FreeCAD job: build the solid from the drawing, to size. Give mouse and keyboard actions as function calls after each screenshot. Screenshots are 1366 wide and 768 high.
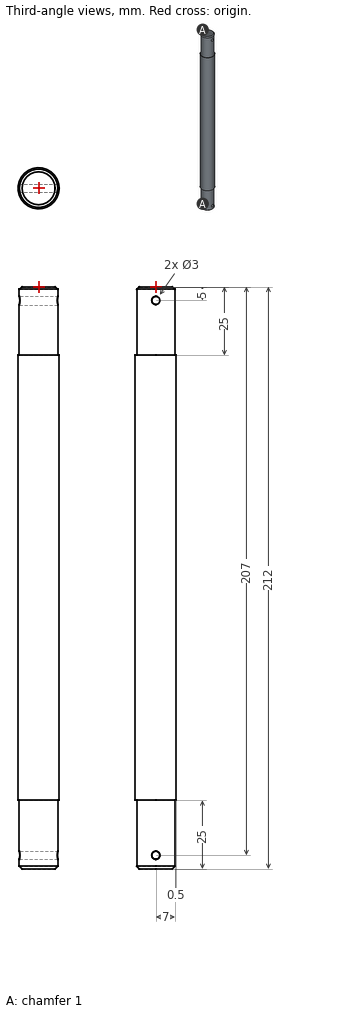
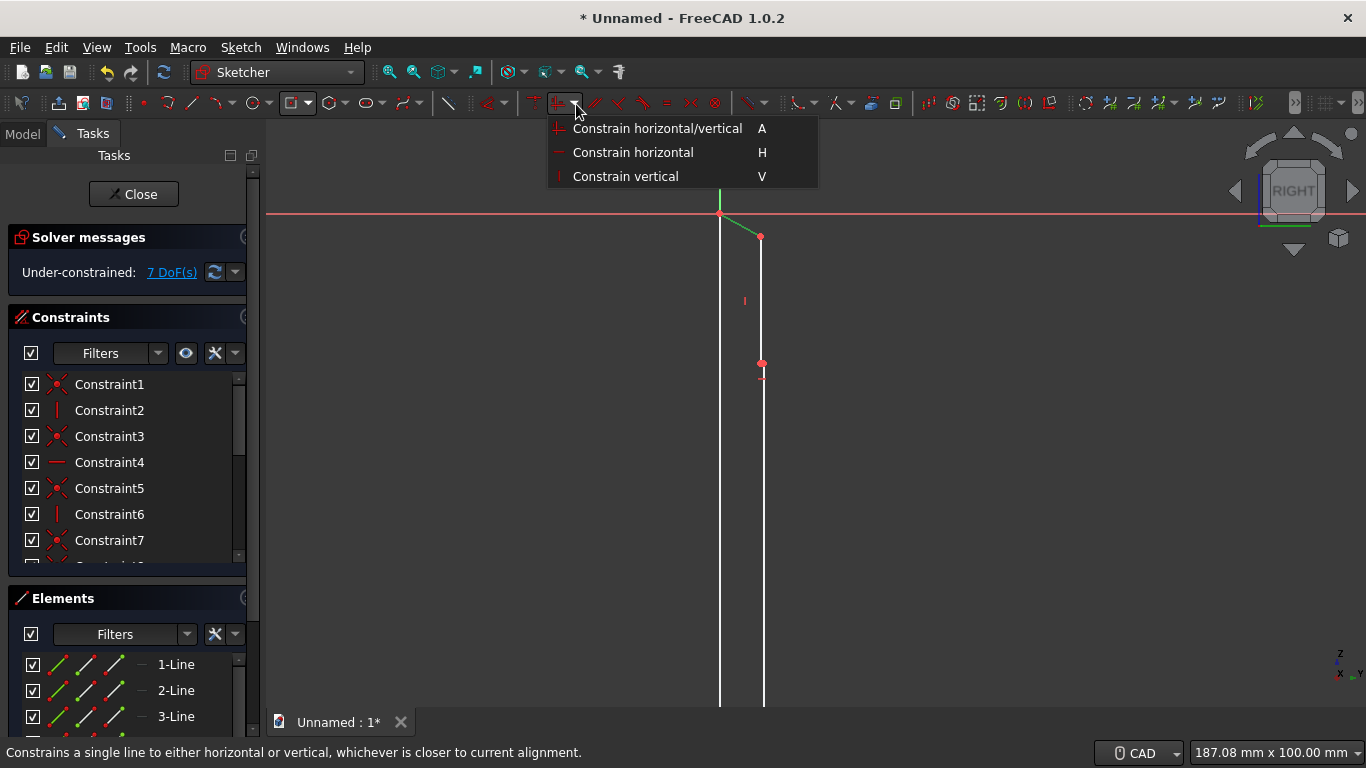
click(683, 152)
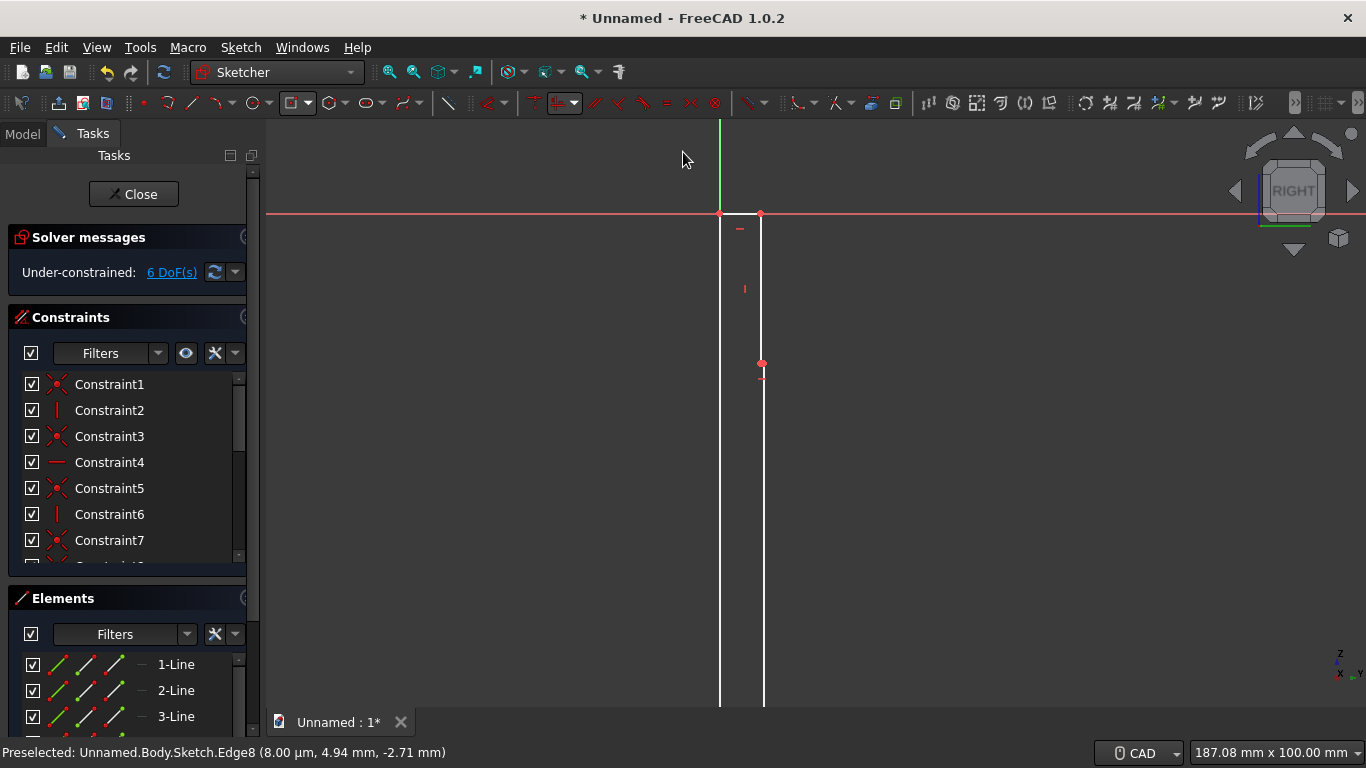
scroll(750, 230, down, 6)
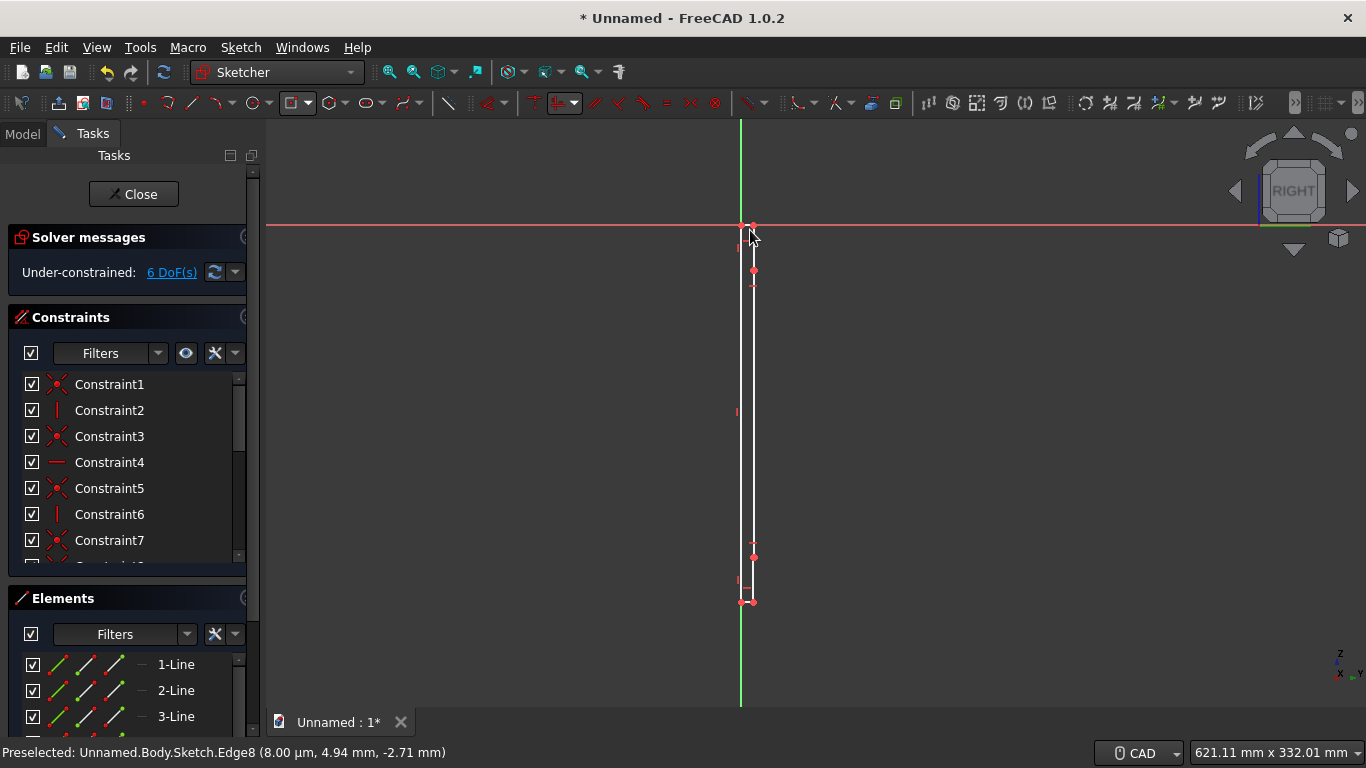
scroll(745, 602, up, 7)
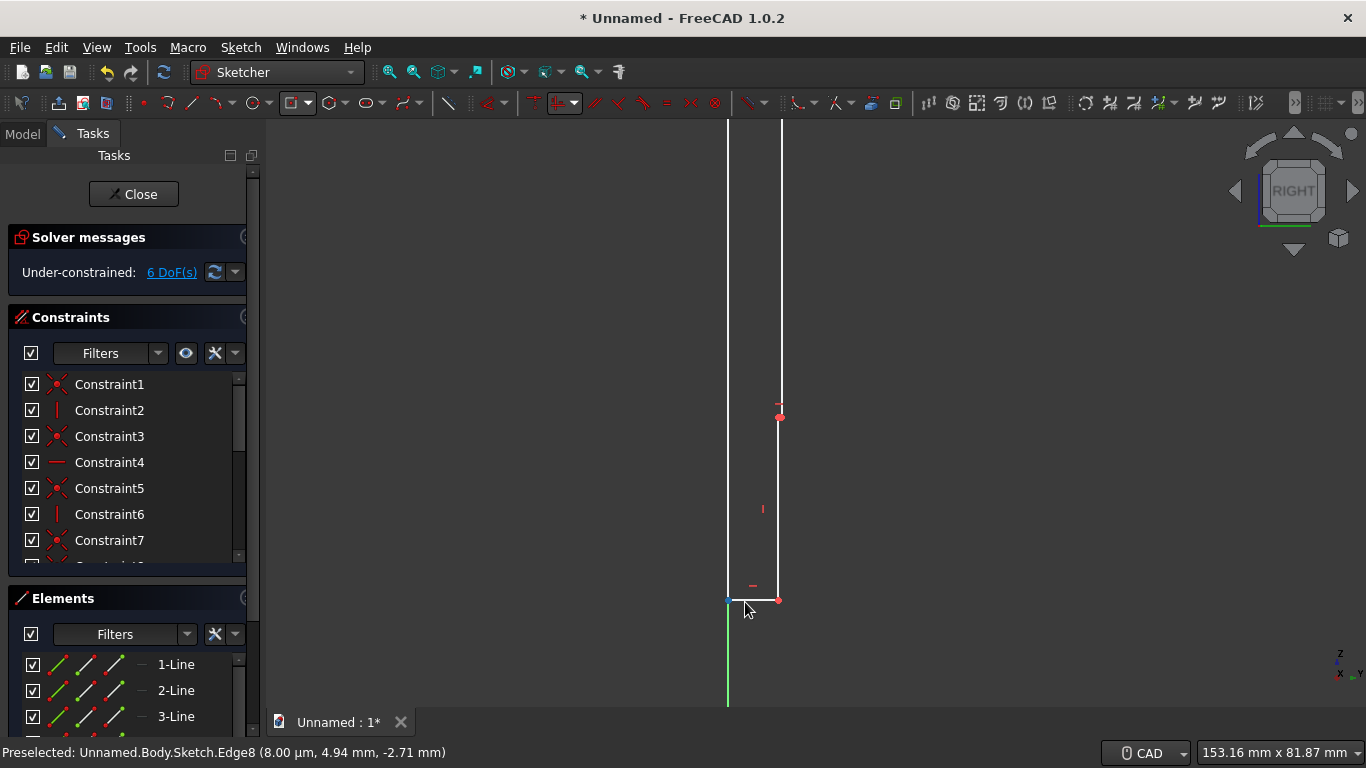
click(743, 600)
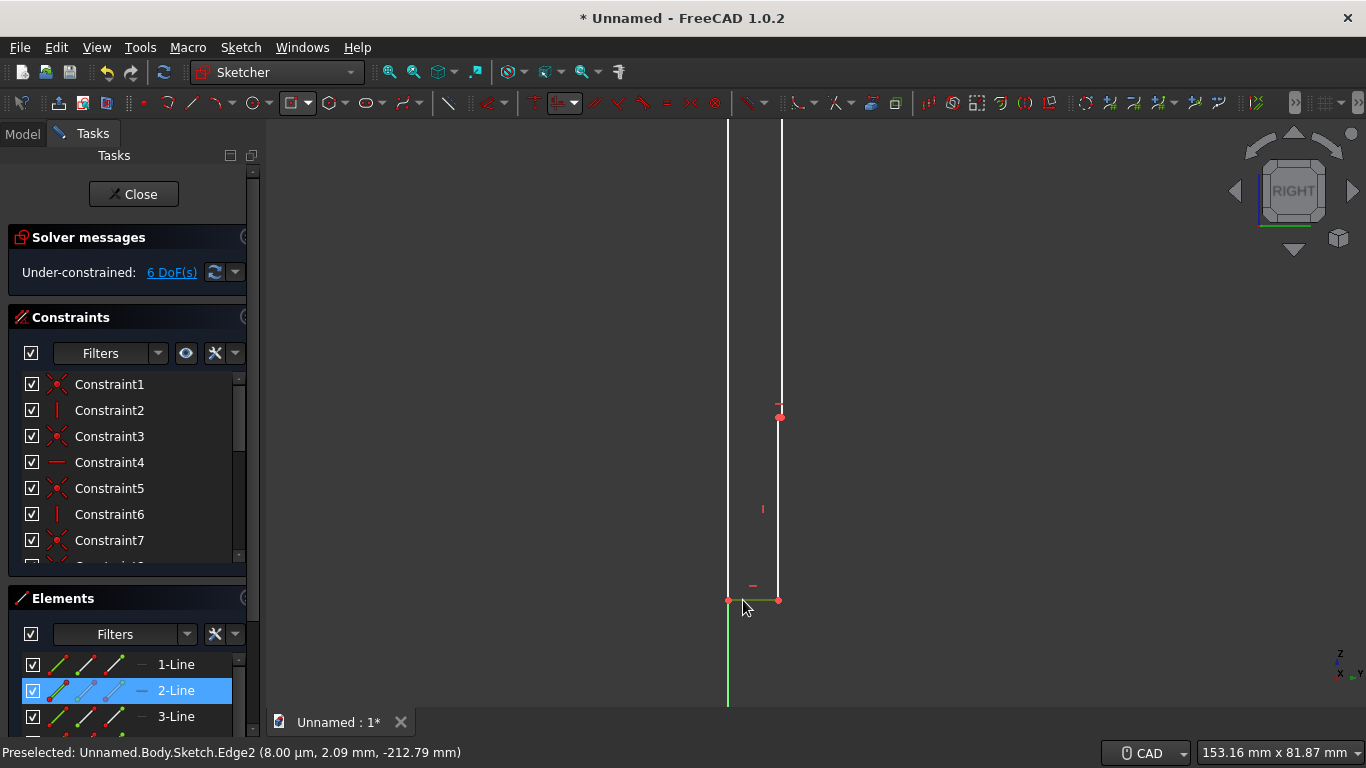
key(l)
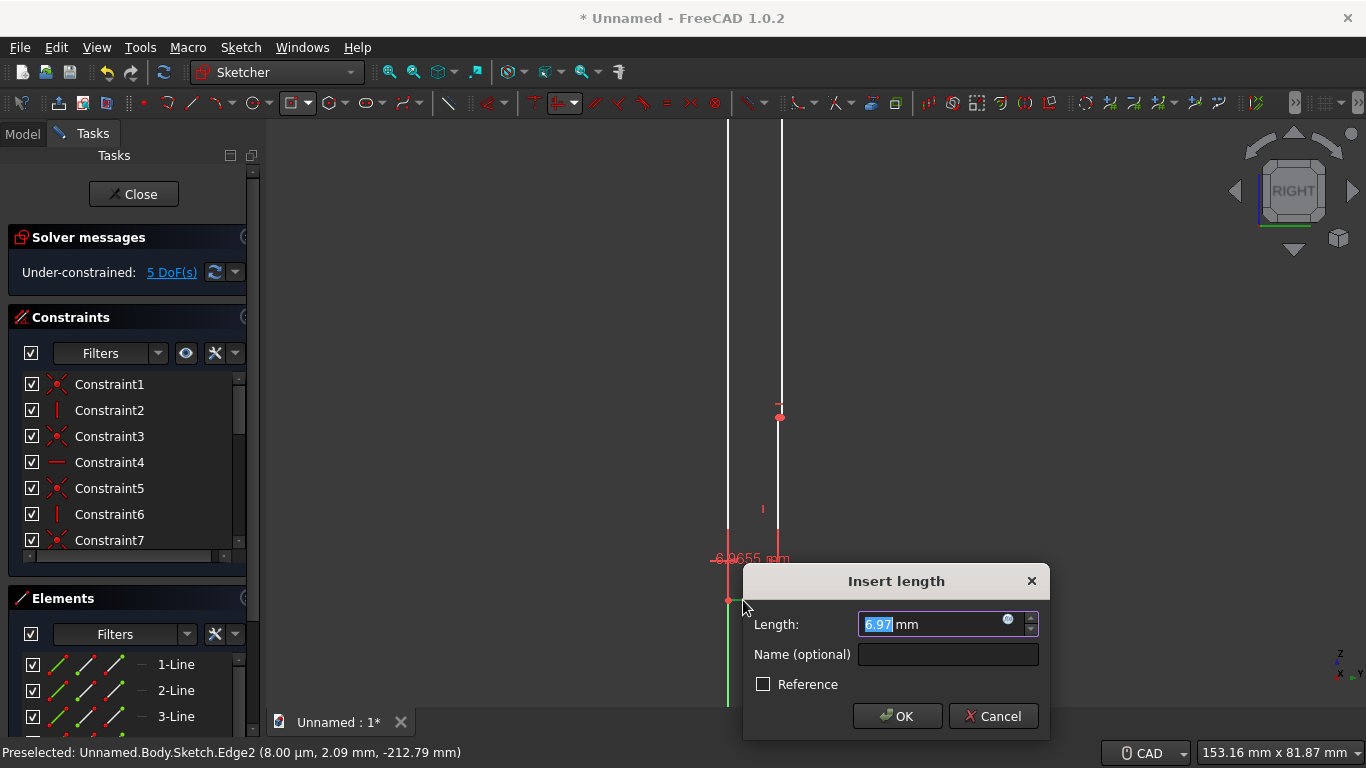
text(7)
key(Return)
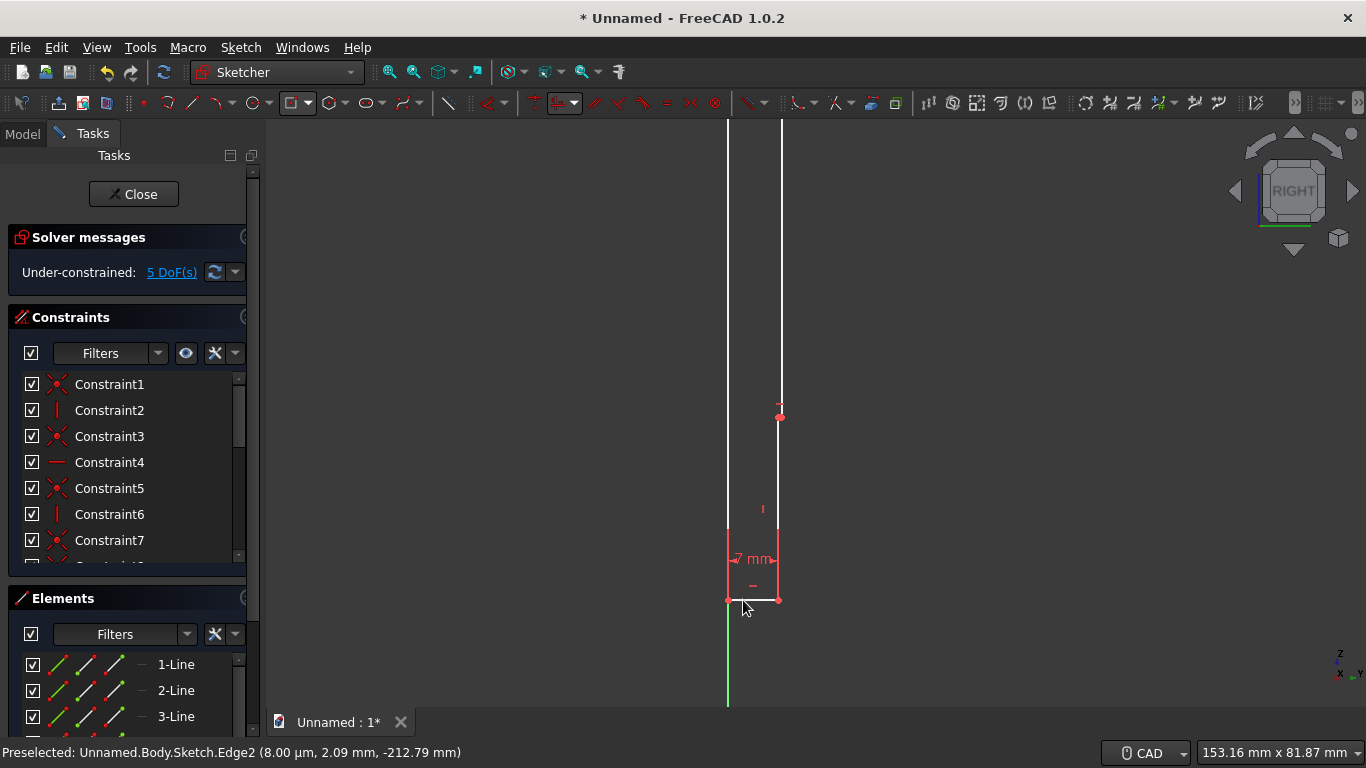
scroll(745, 603, down, 7)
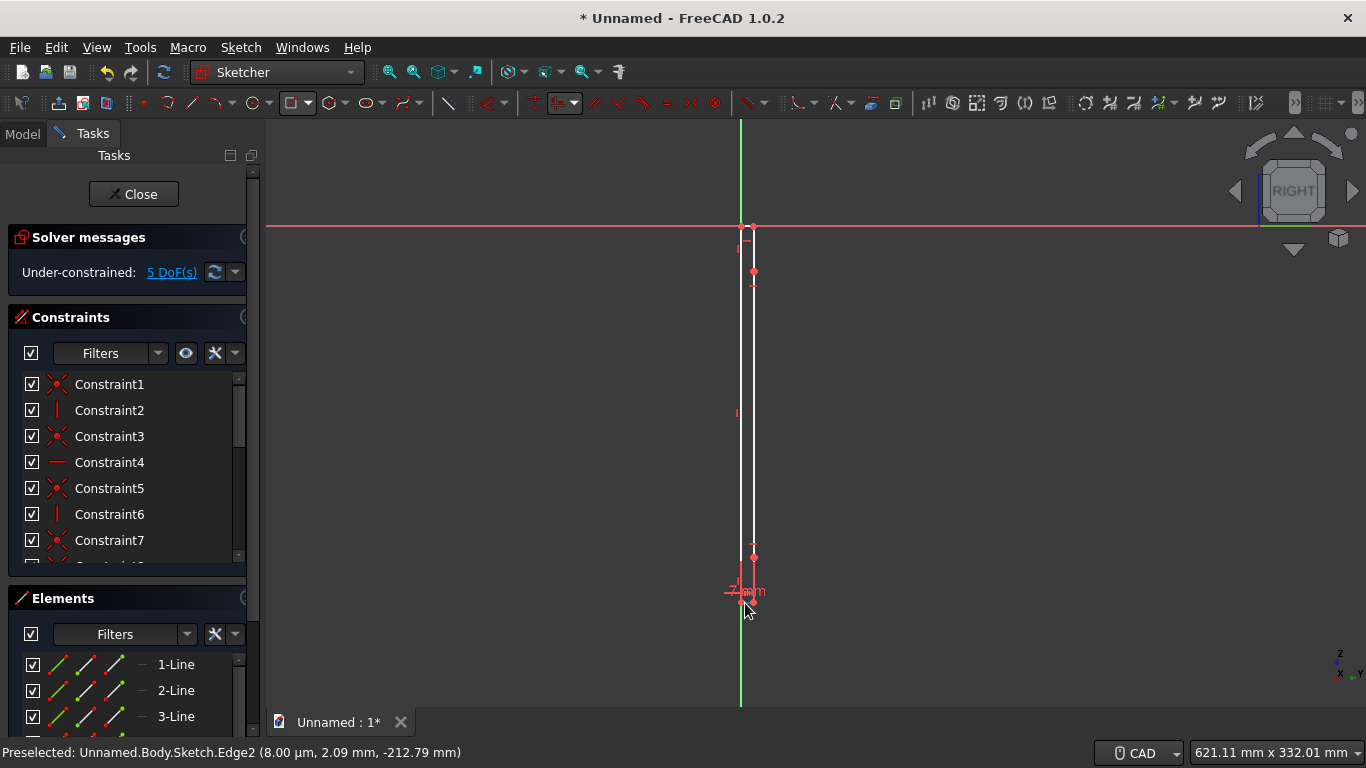
scroll(750, 226, up, 7)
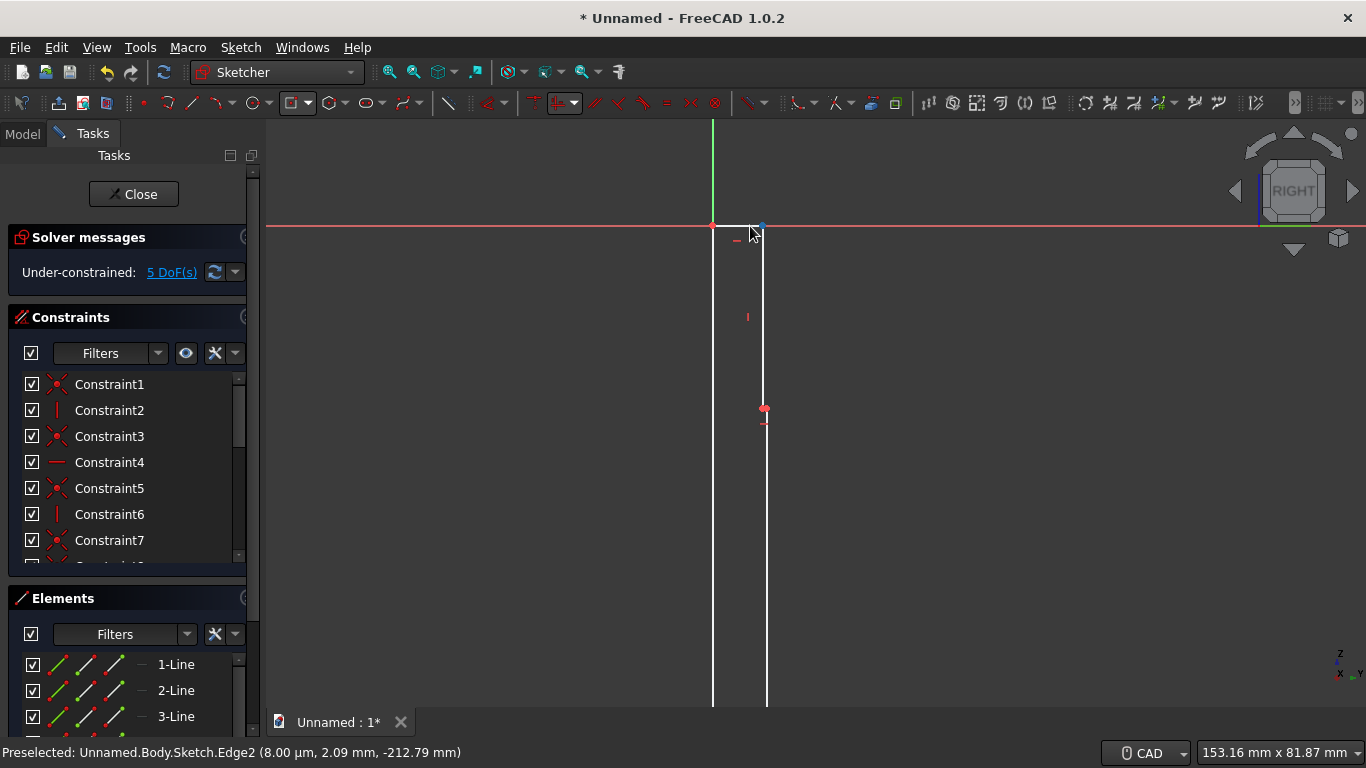
click(748, 226)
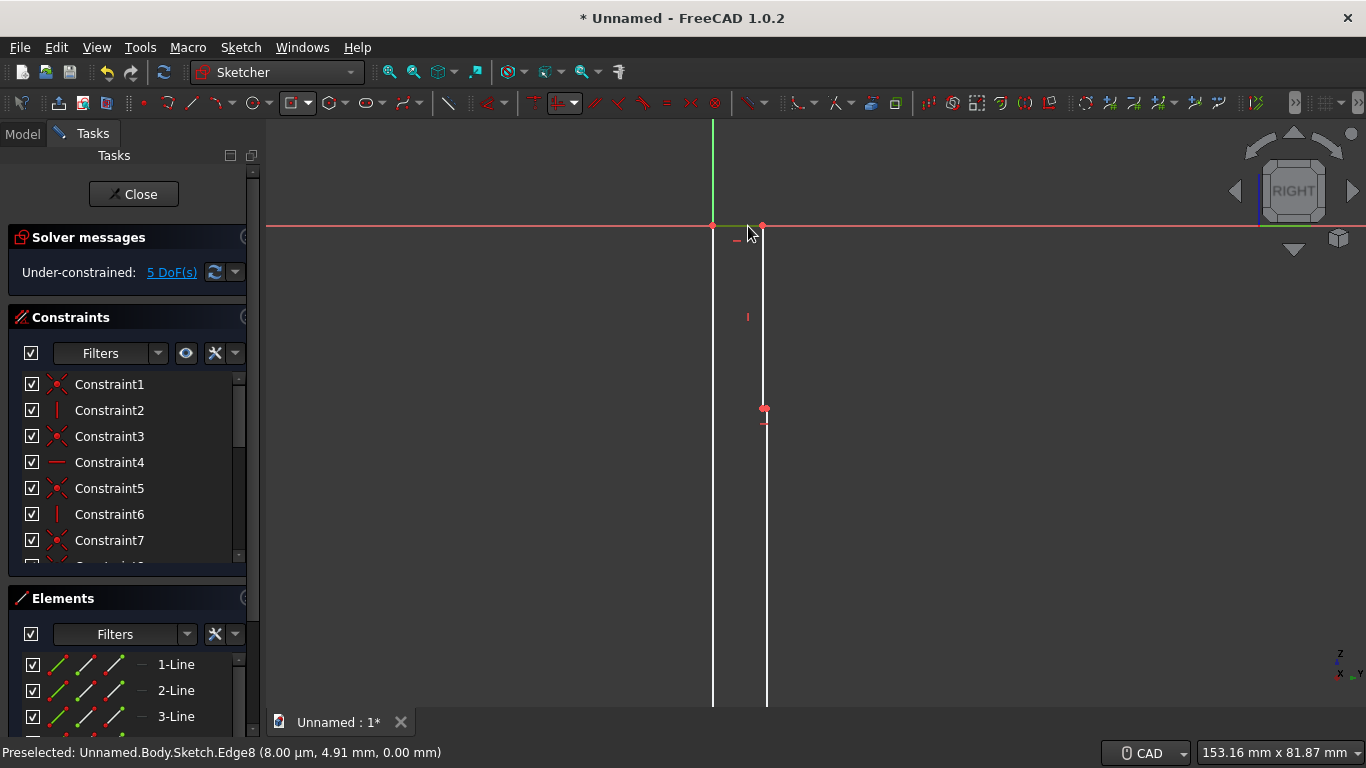
key(l)